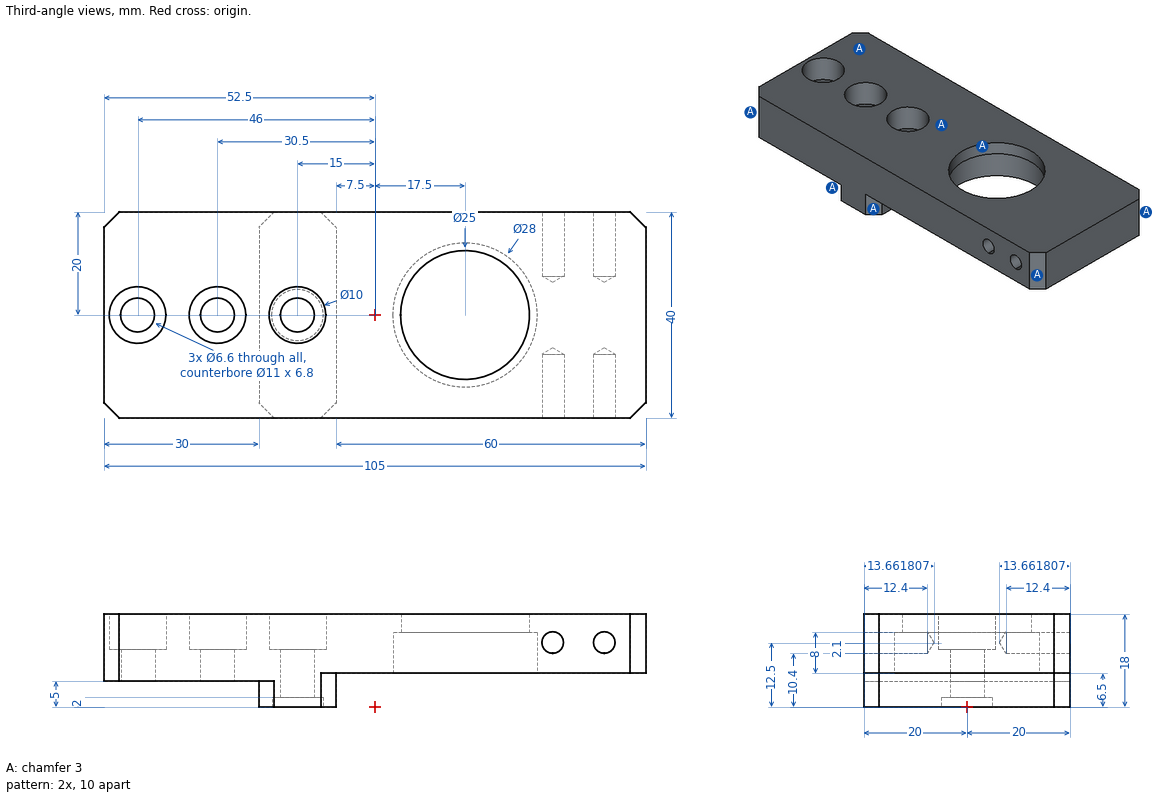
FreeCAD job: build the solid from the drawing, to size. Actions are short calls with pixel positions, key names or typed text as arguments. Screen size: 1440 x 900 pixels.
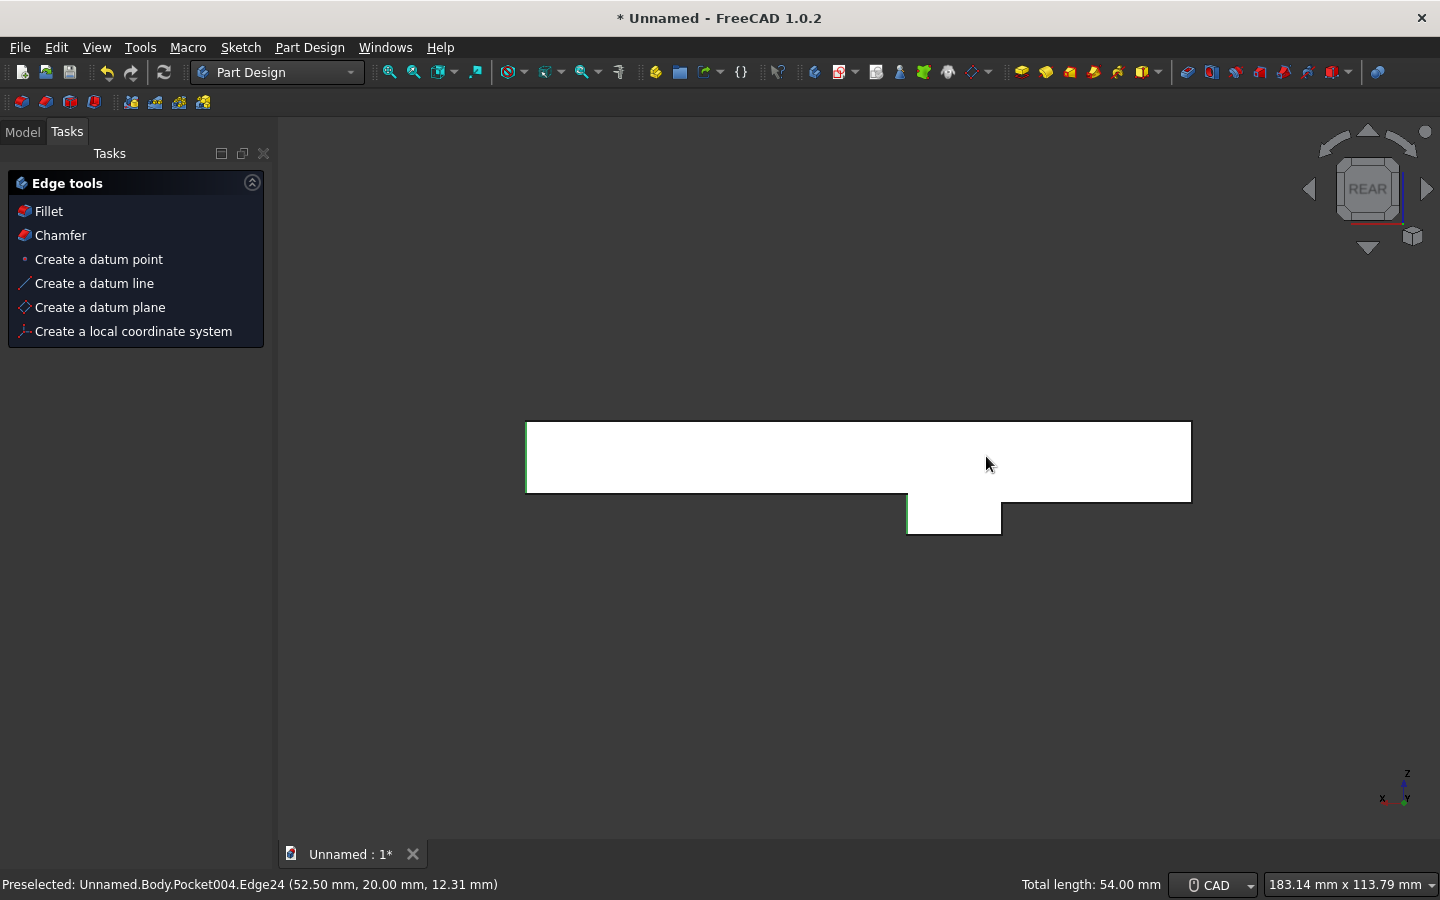
click(1002, 518, ctrl)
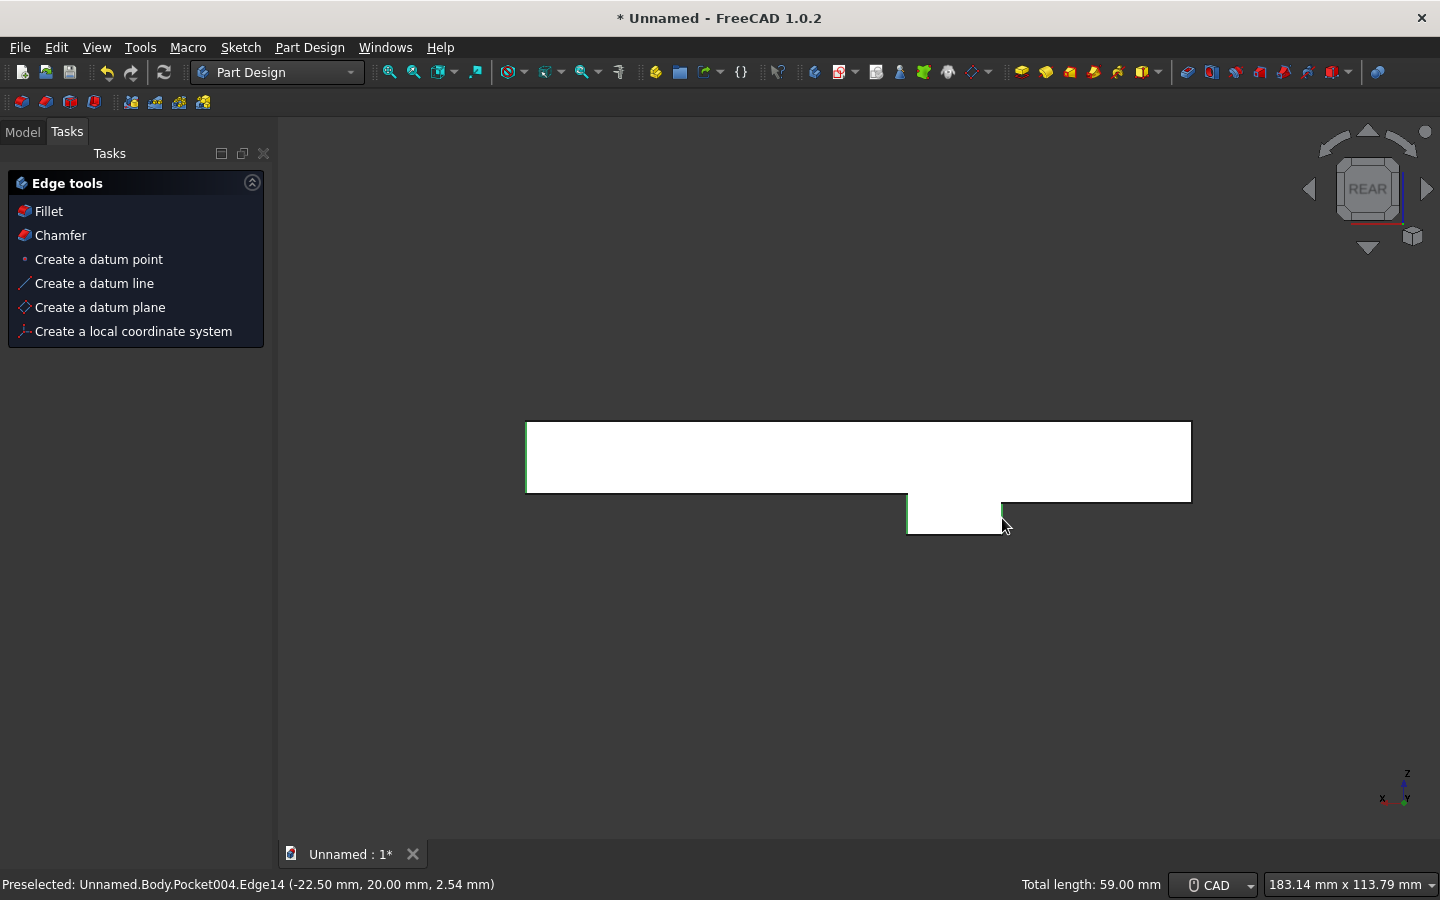
click(1192, 461, ctrl)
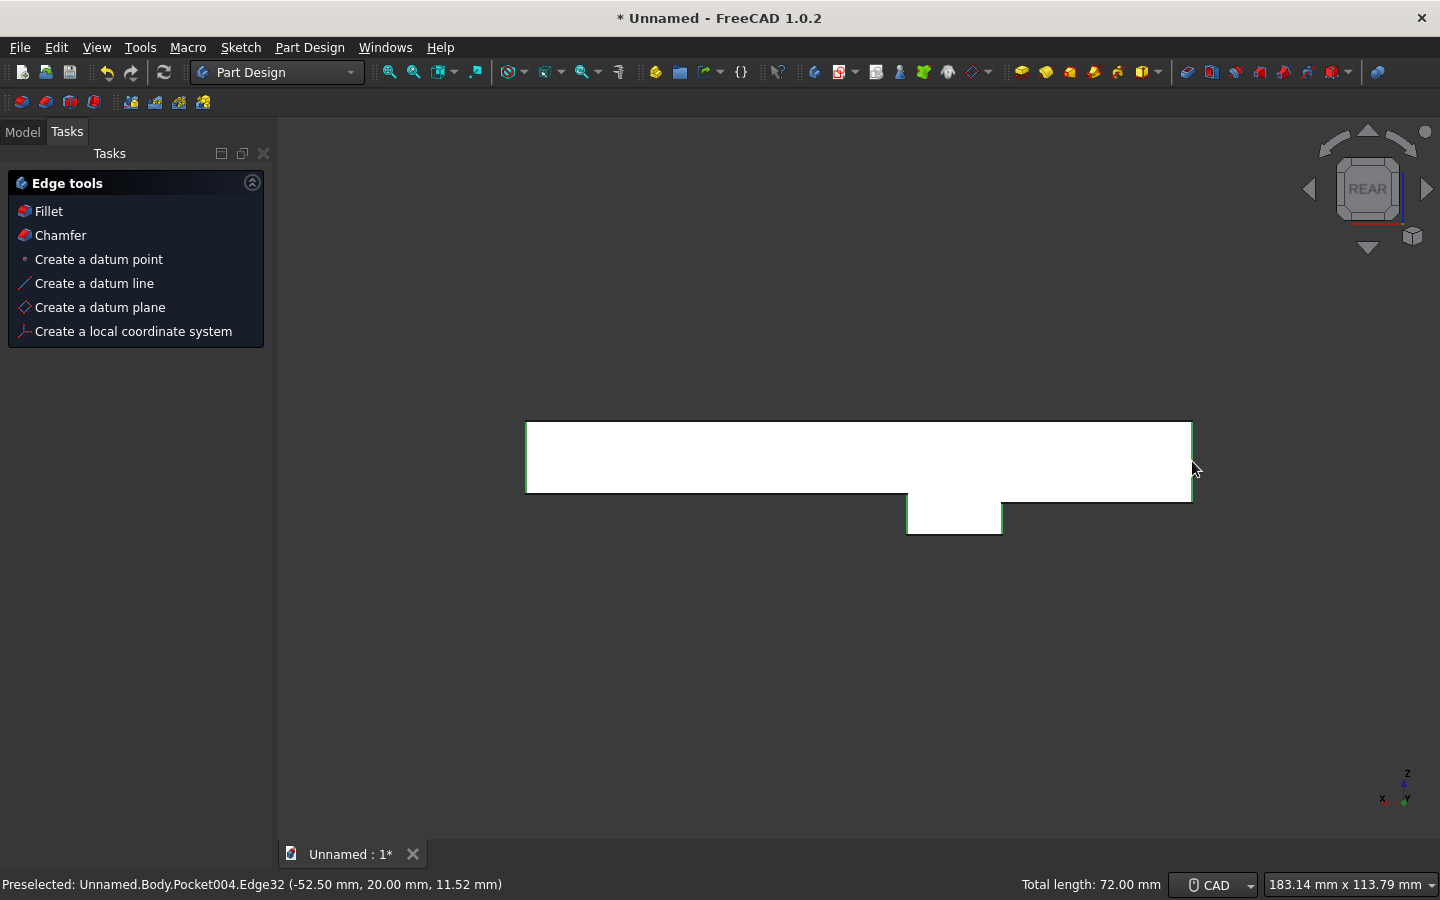
click(46, 102)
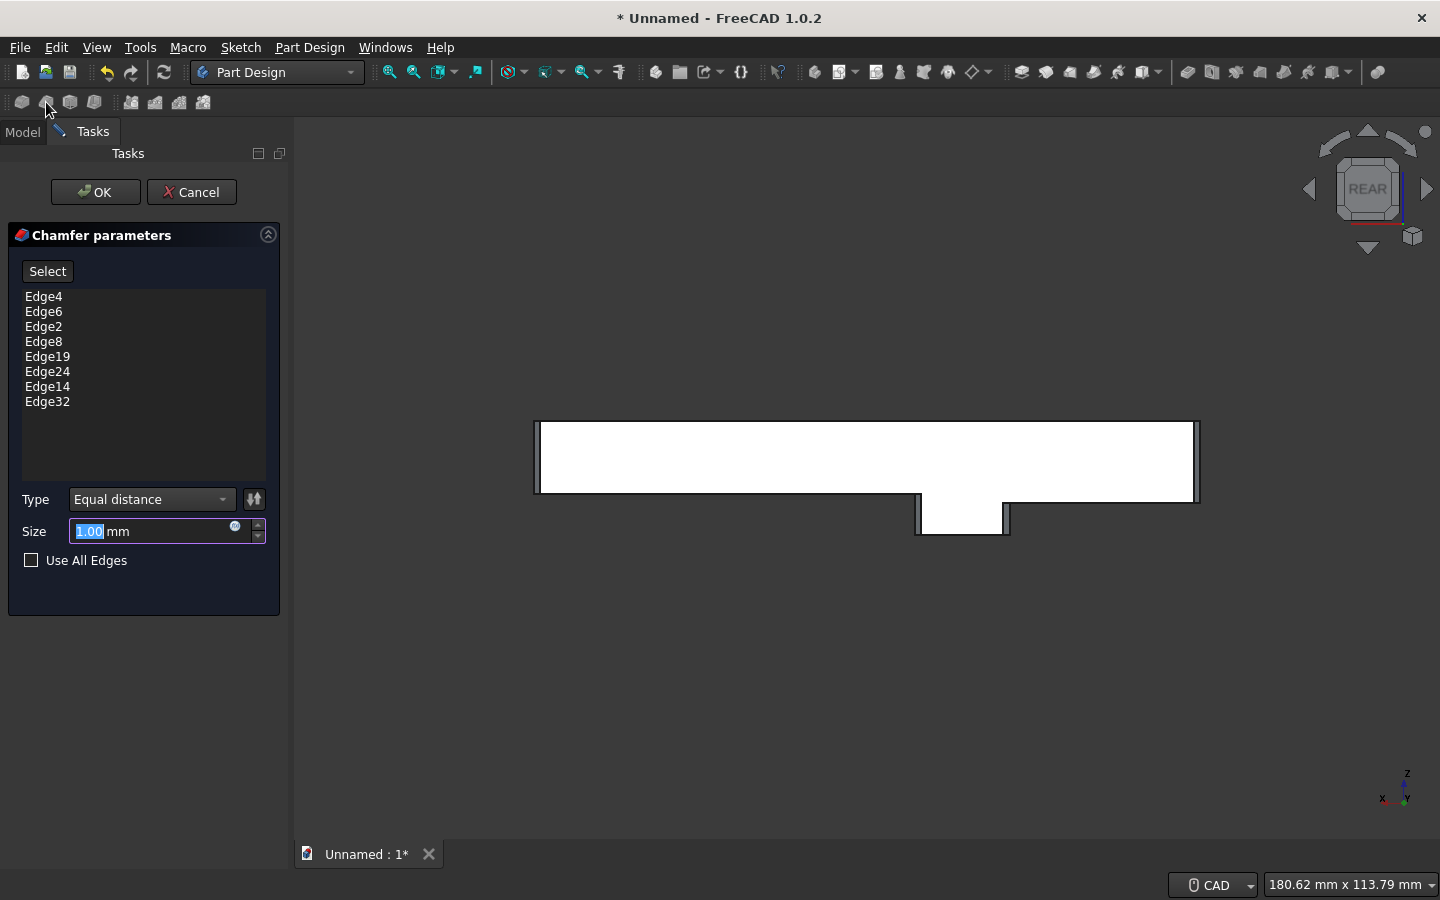
text(3)
key(Tab)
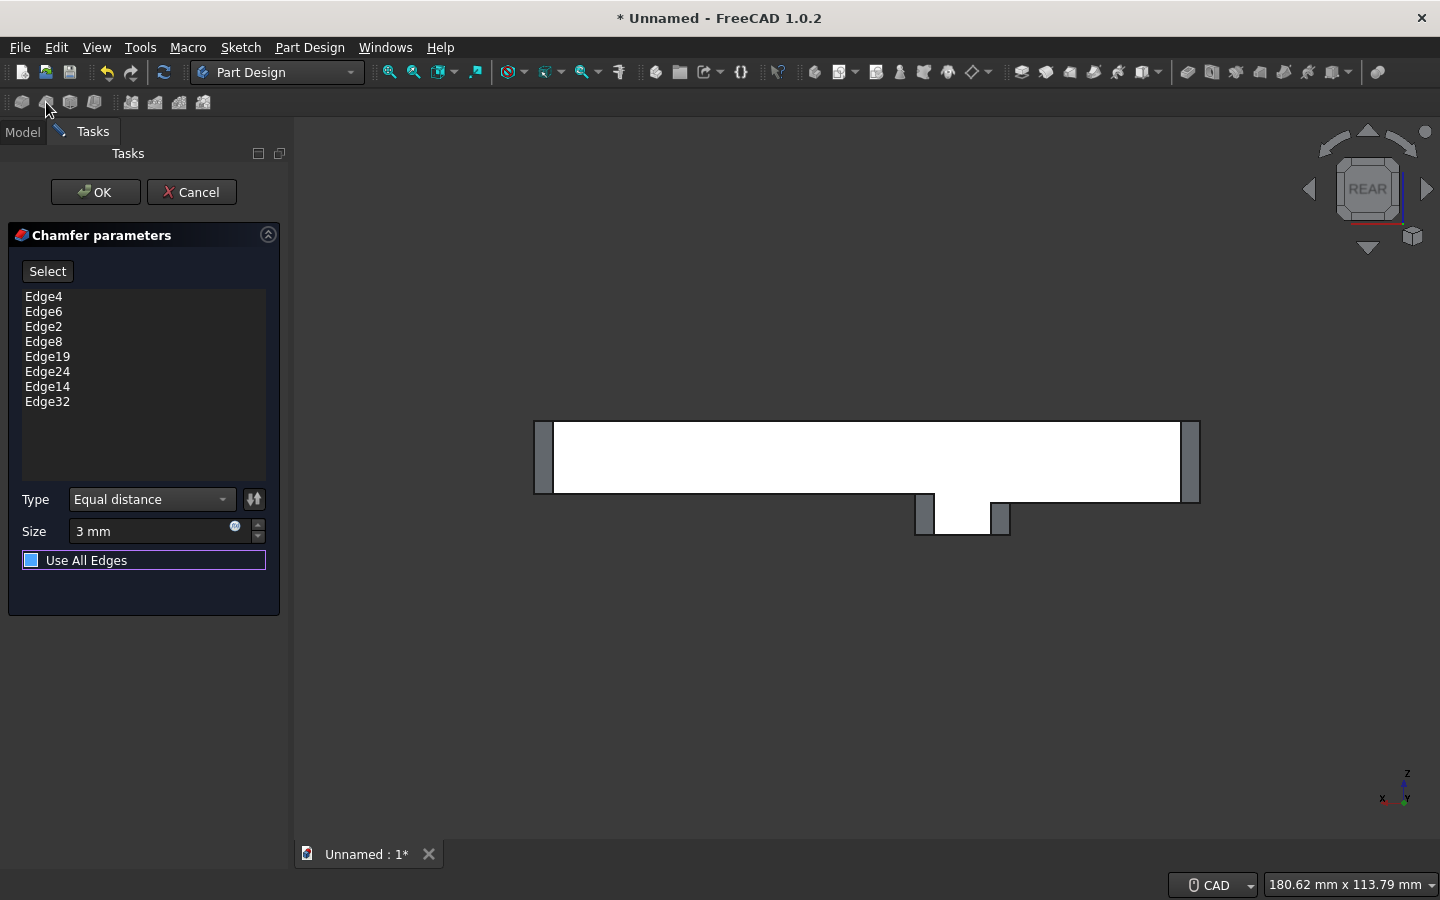
click(96, 192)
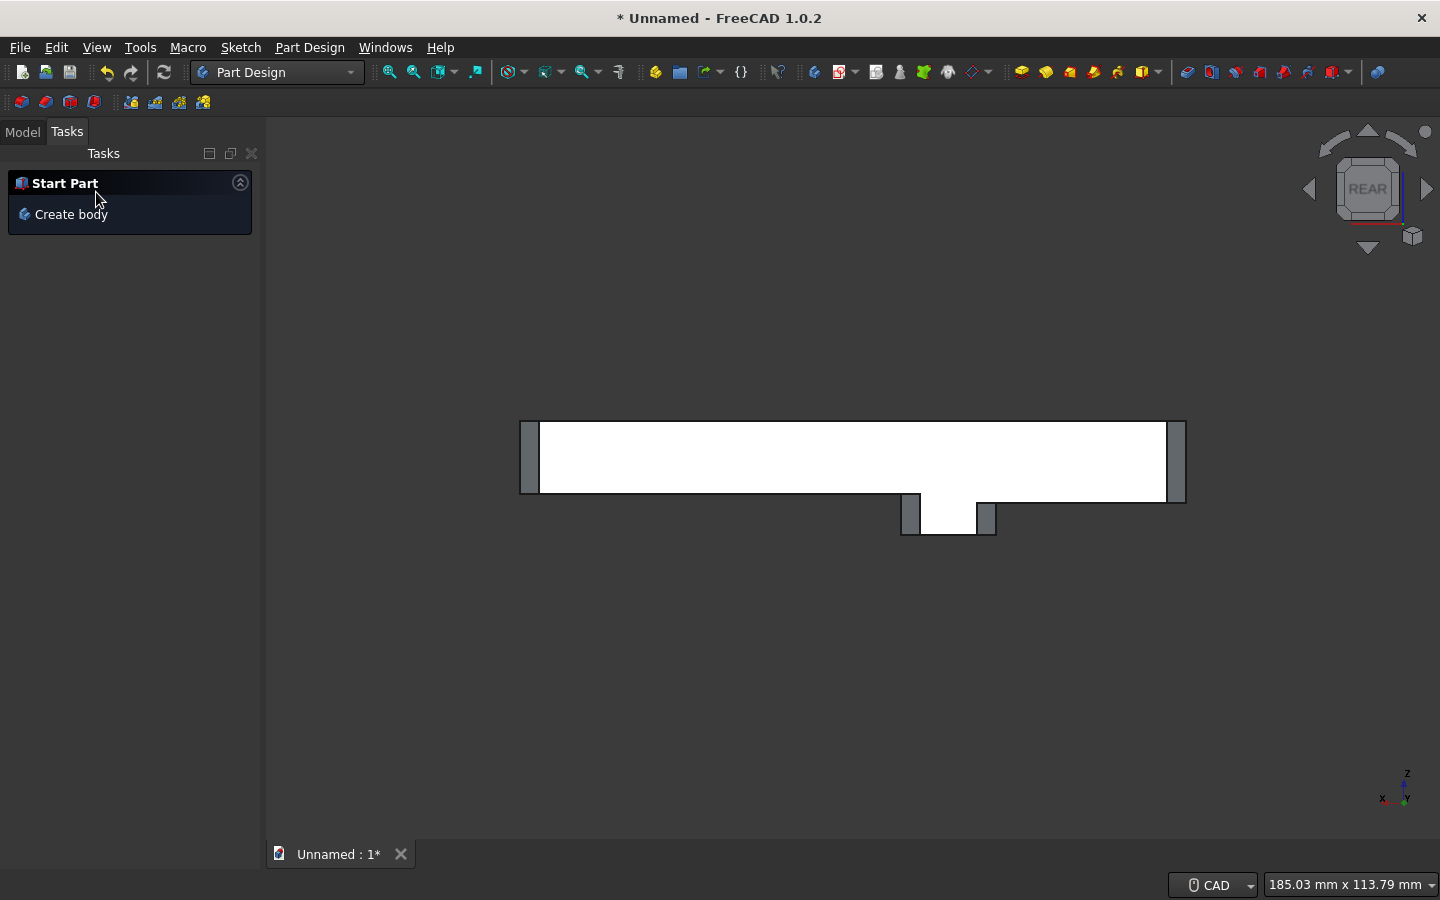
click(23, 131)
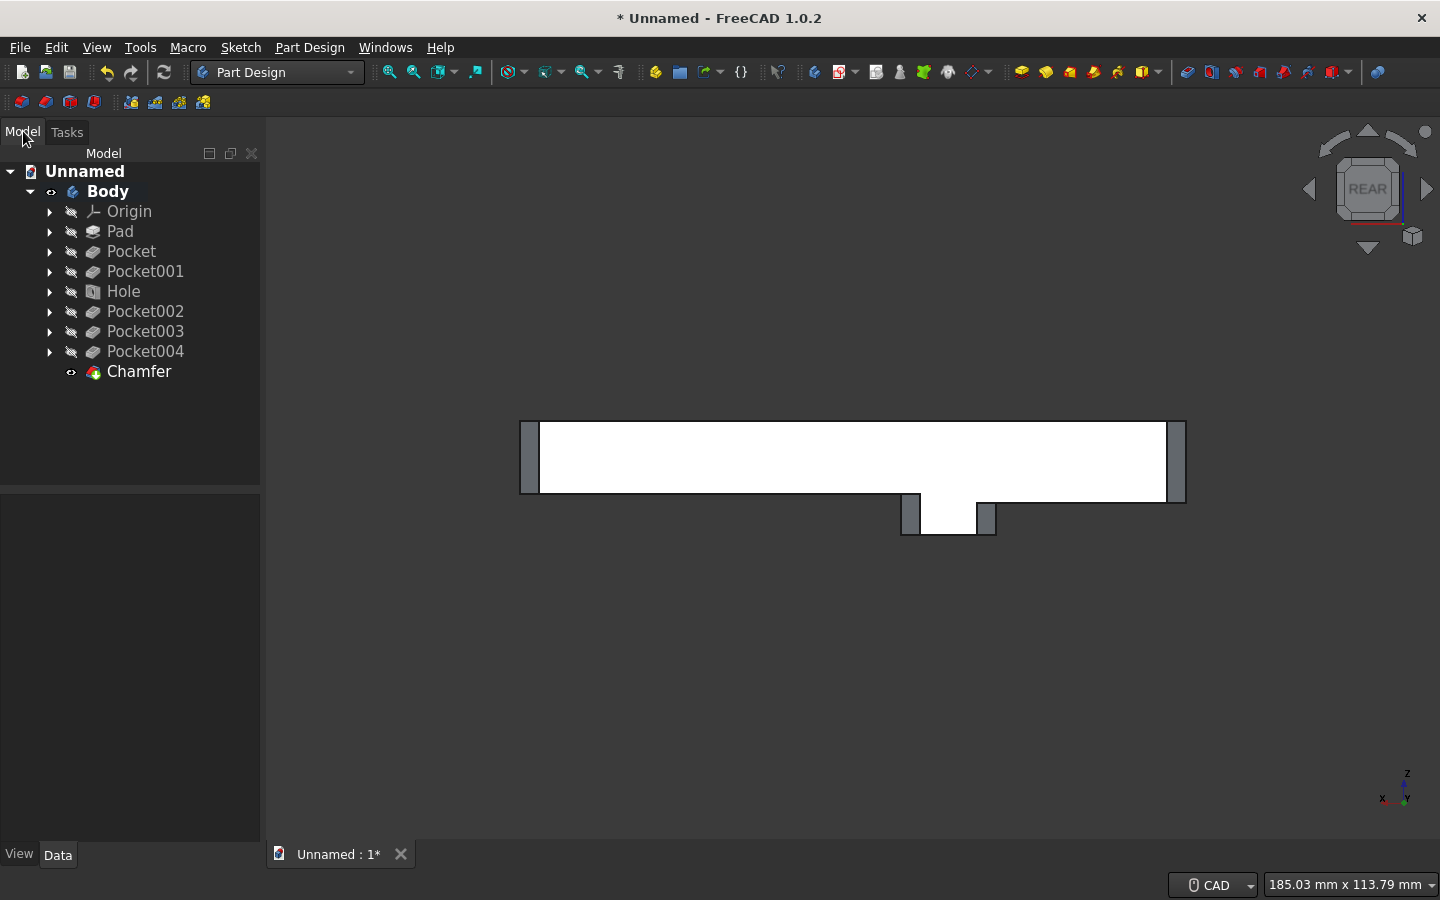
click(50, 212)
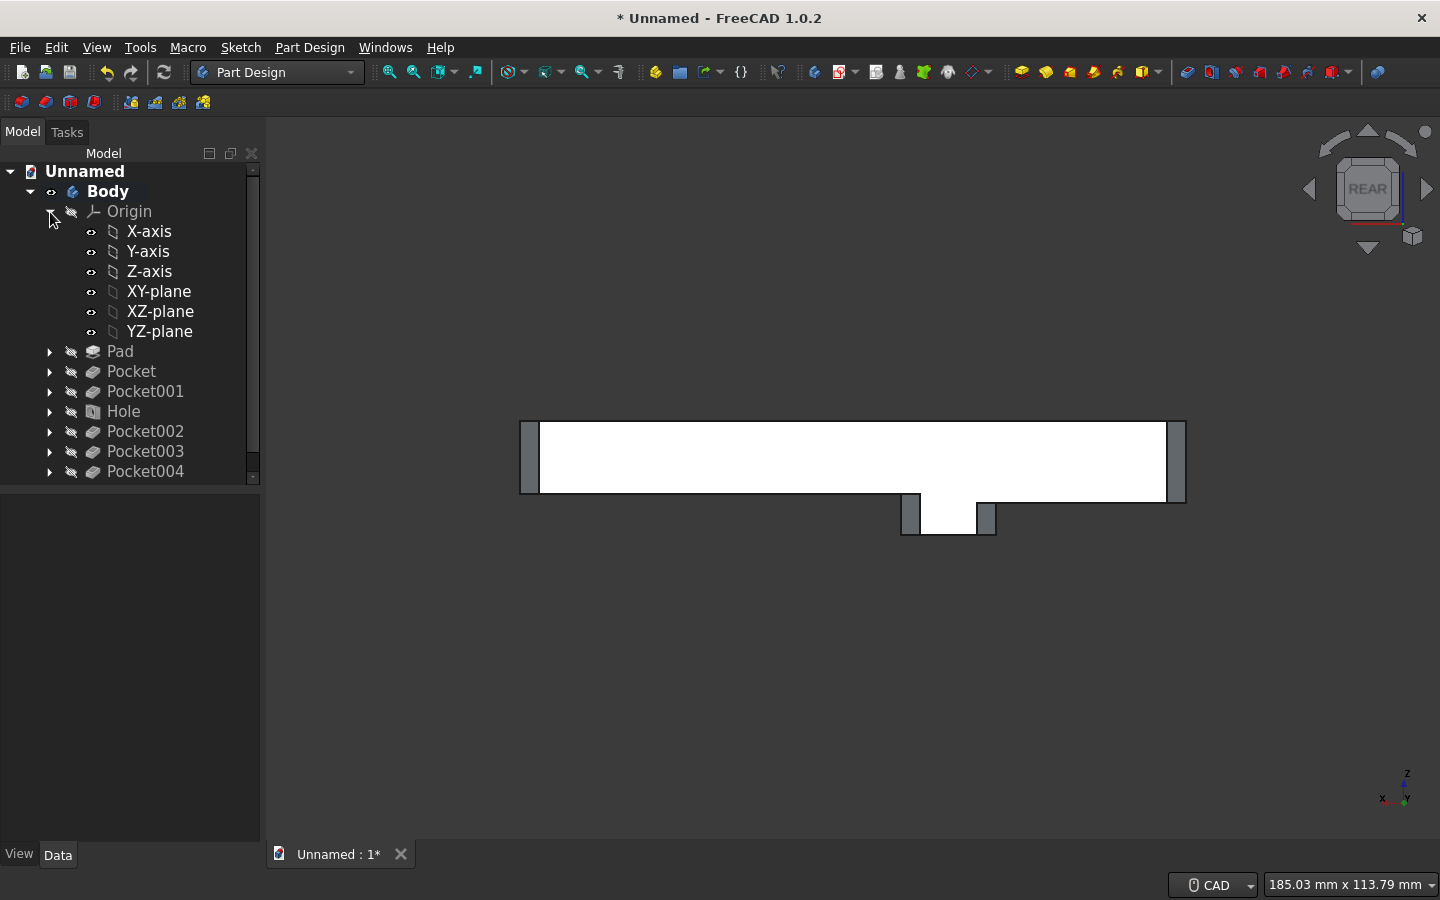
click(136, 332)